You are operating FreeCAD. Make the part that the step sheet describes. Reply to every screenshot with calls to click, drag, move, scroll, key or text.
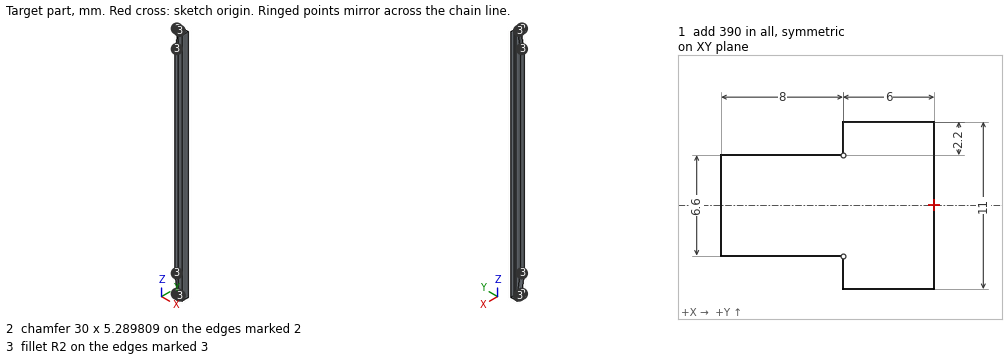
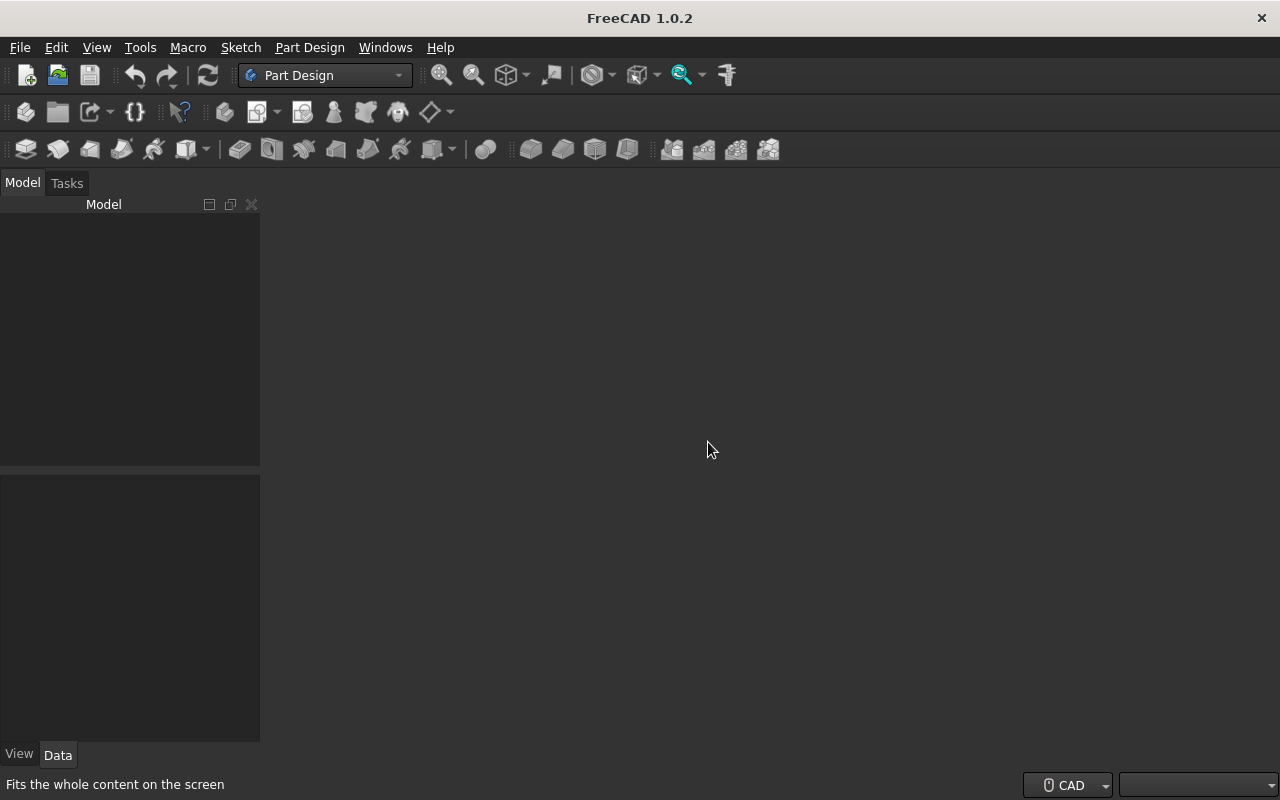
click(26, 76)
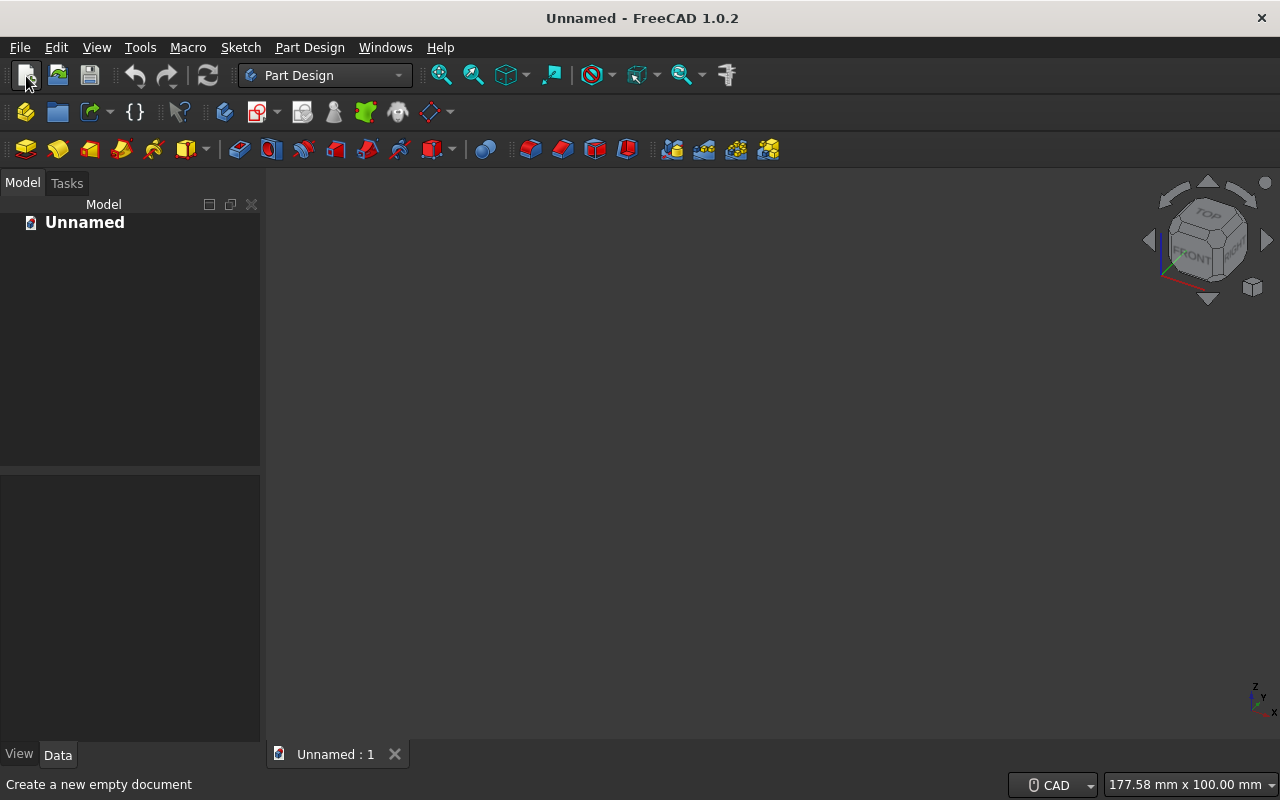
click(258, 112)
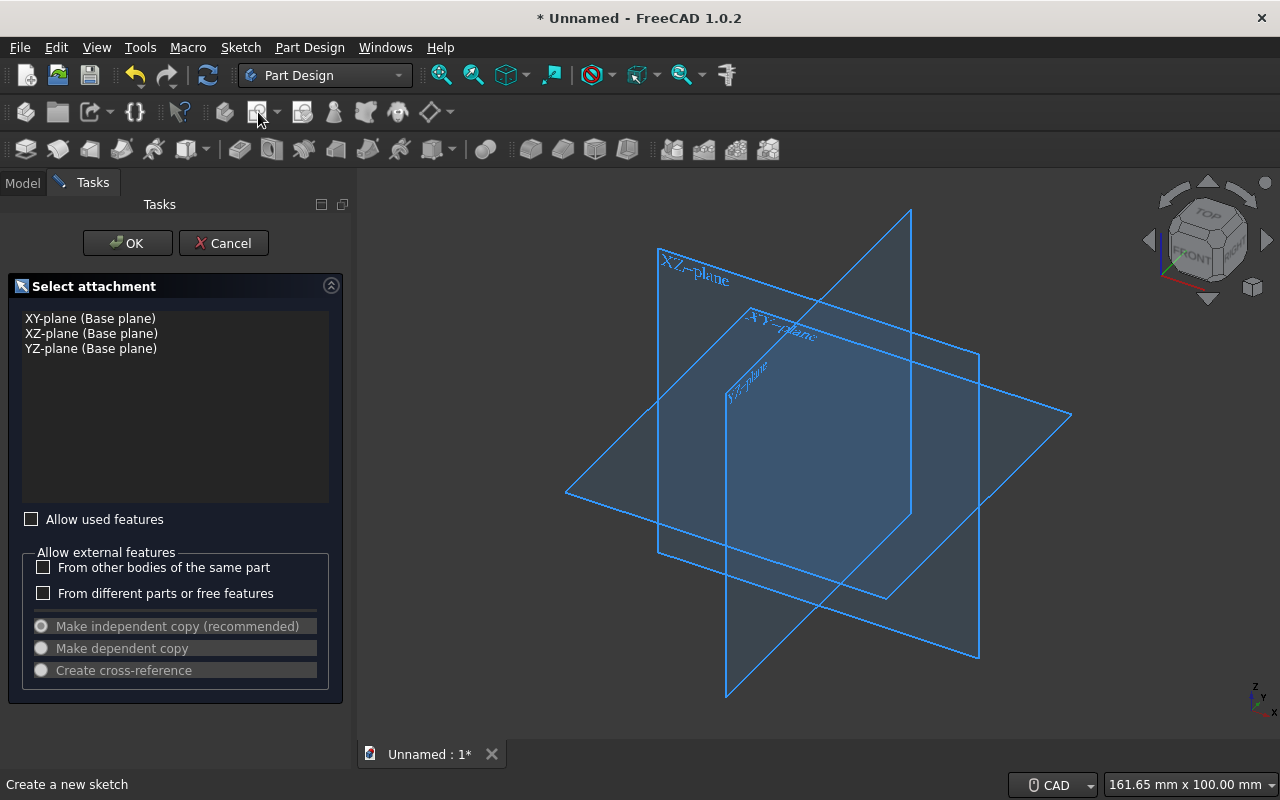
click(82, 318)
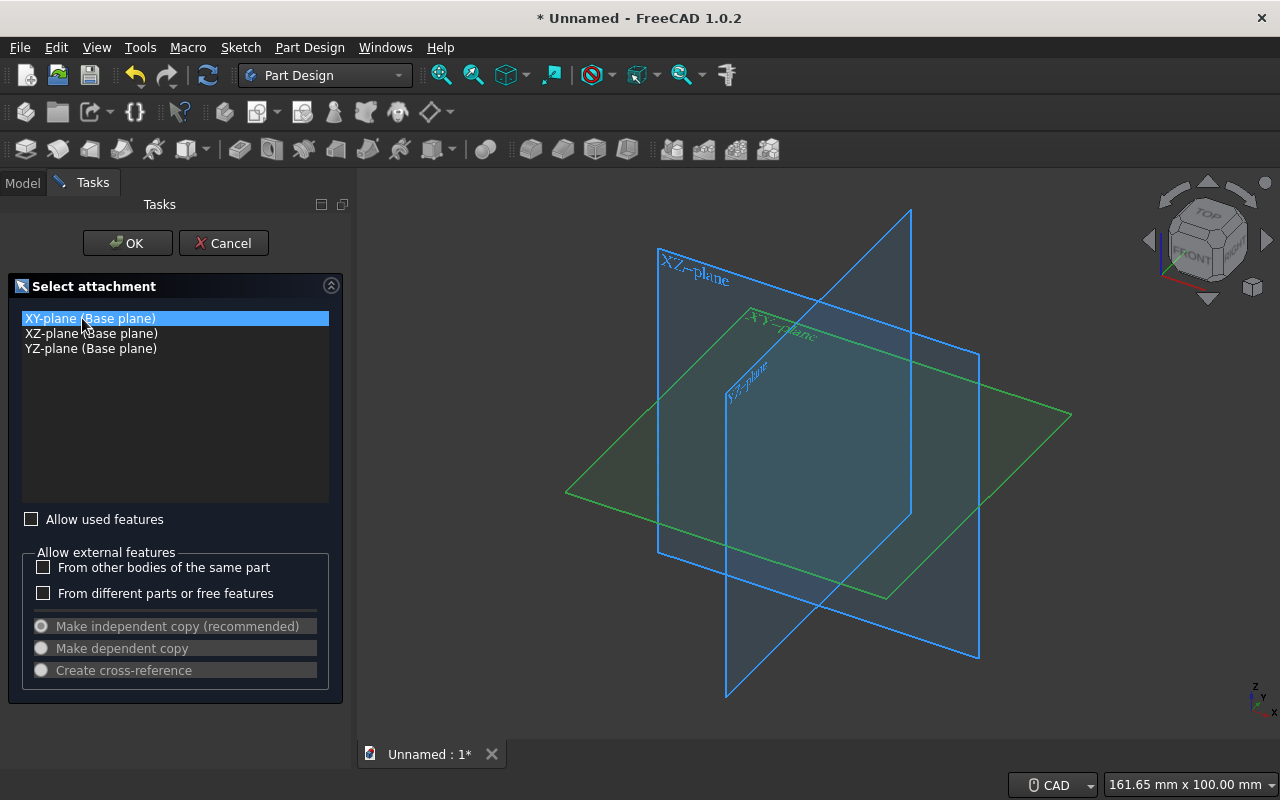
click(128, 243)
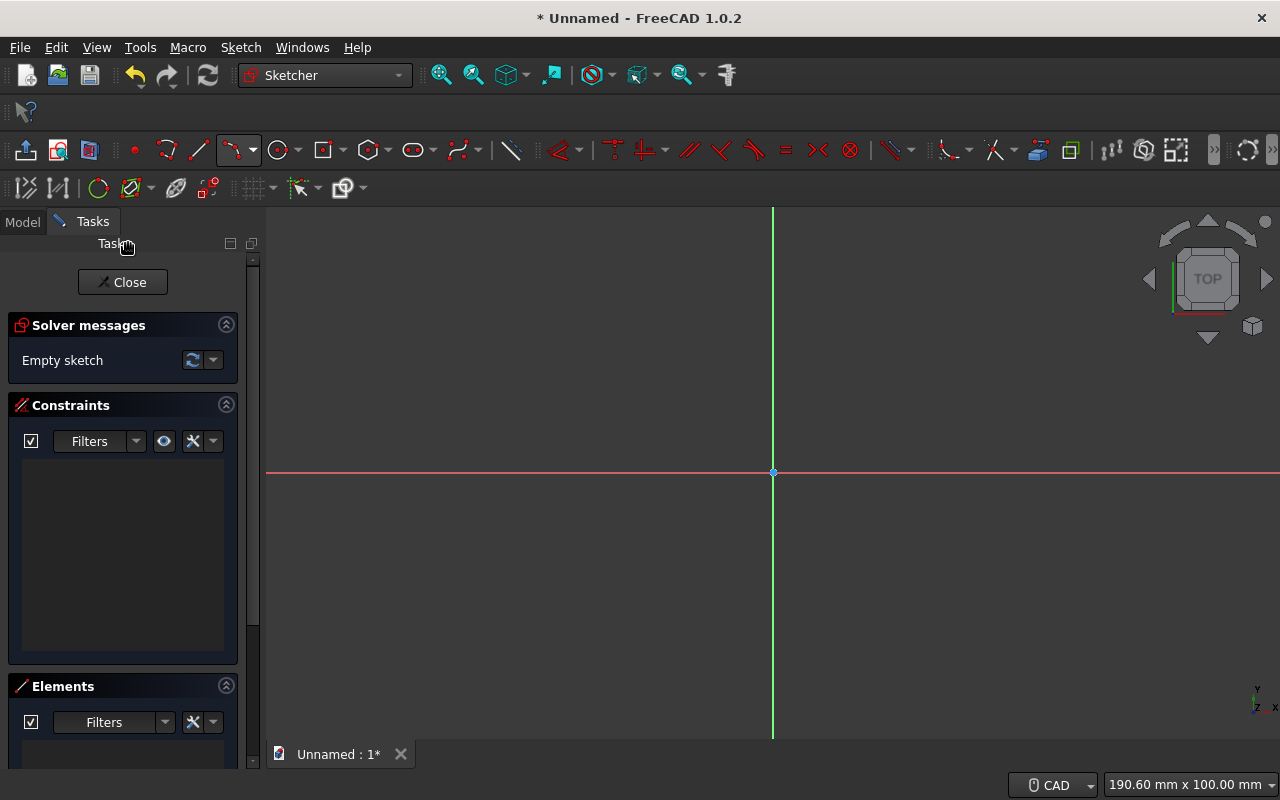
scroll(742, 473, up, 9)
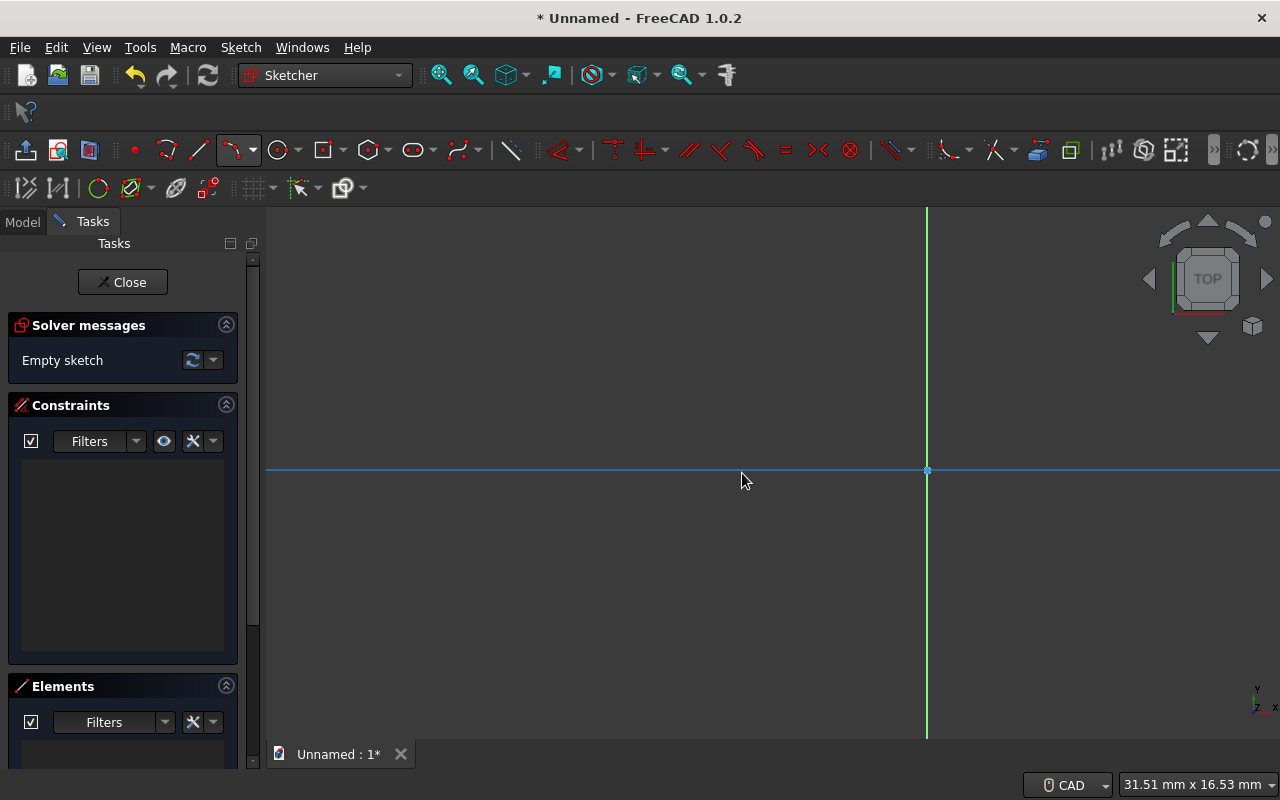
click(168, 150)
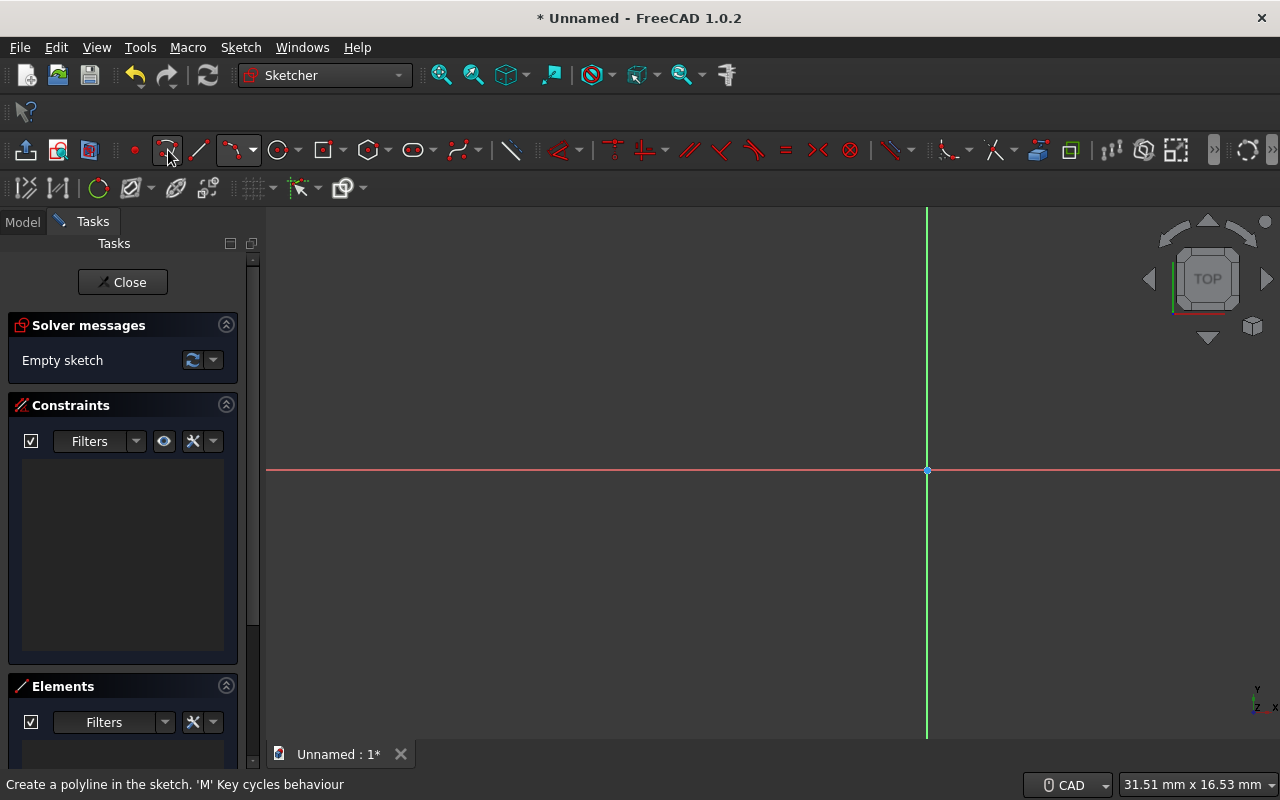
click(927, 647)
click(918, 293)
click(734, 293)
click(734, 364)
click(477, 364)
click(477, 577)
click(734, 577)
click(734, 647)
click(927, 648)
key(Escape)
key(Escape)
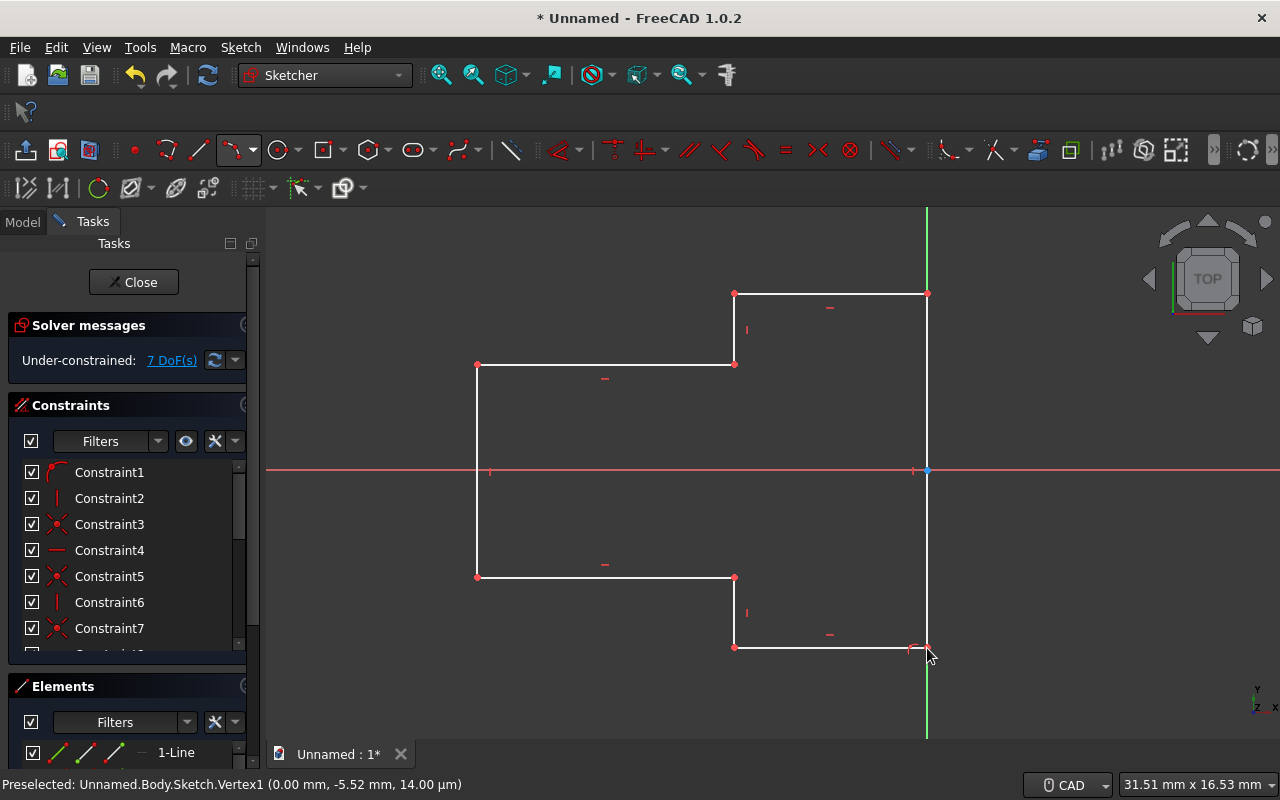
click(734, 365)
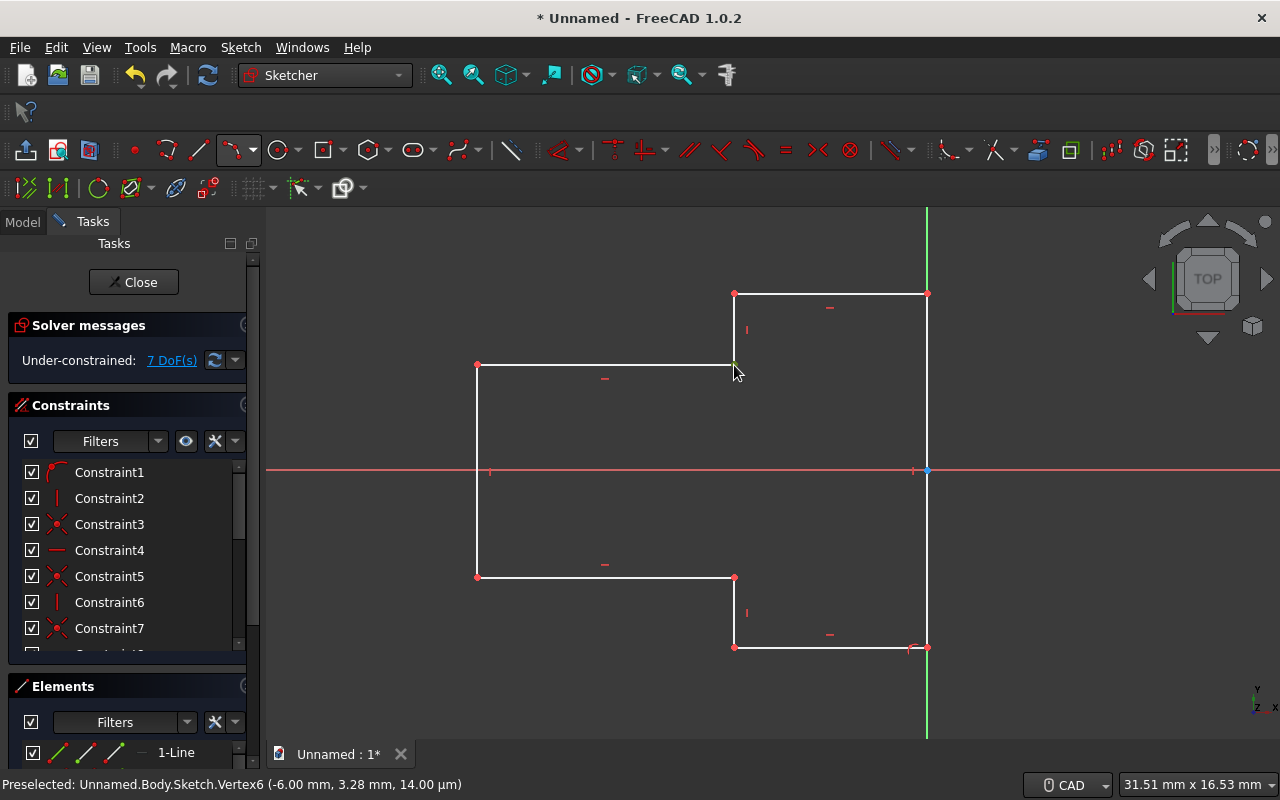
click(734, 578)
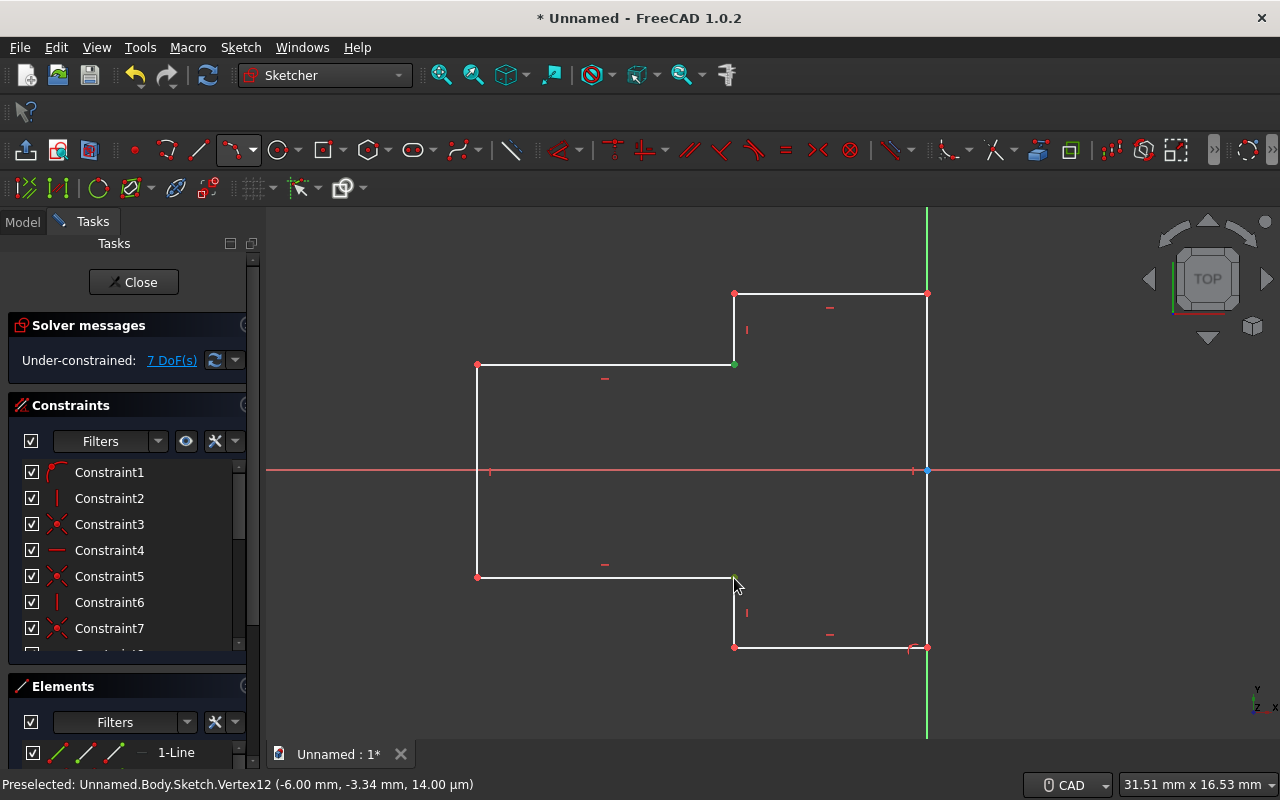
click(353, 470)